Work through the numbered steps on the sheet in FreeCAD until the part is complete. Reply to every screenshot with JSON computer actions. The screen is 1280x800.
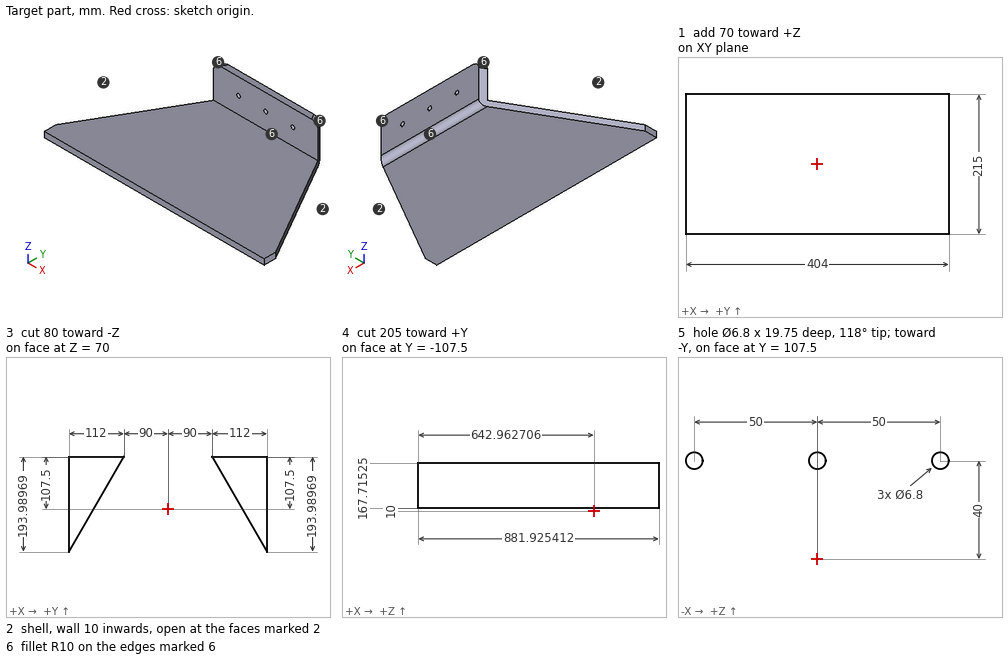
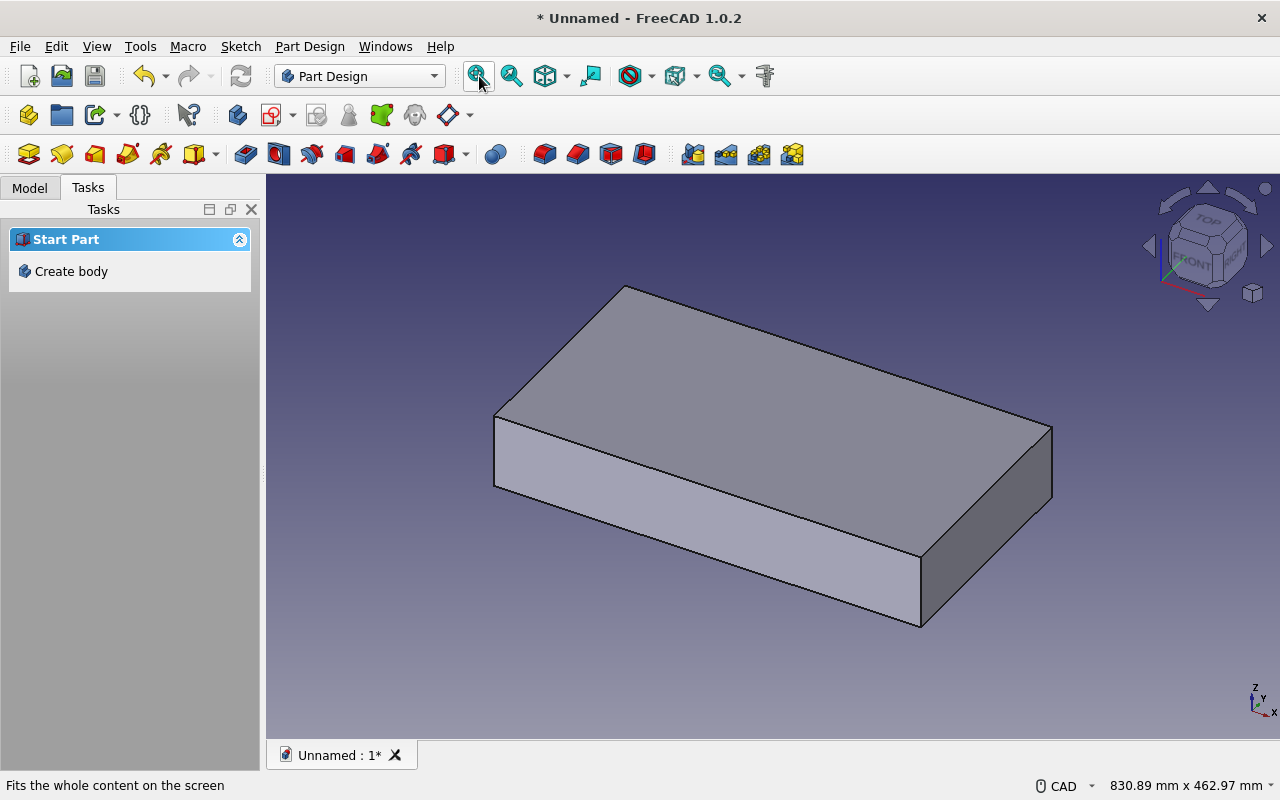
{"action": "left_click", "coordinate": [1024, 489]}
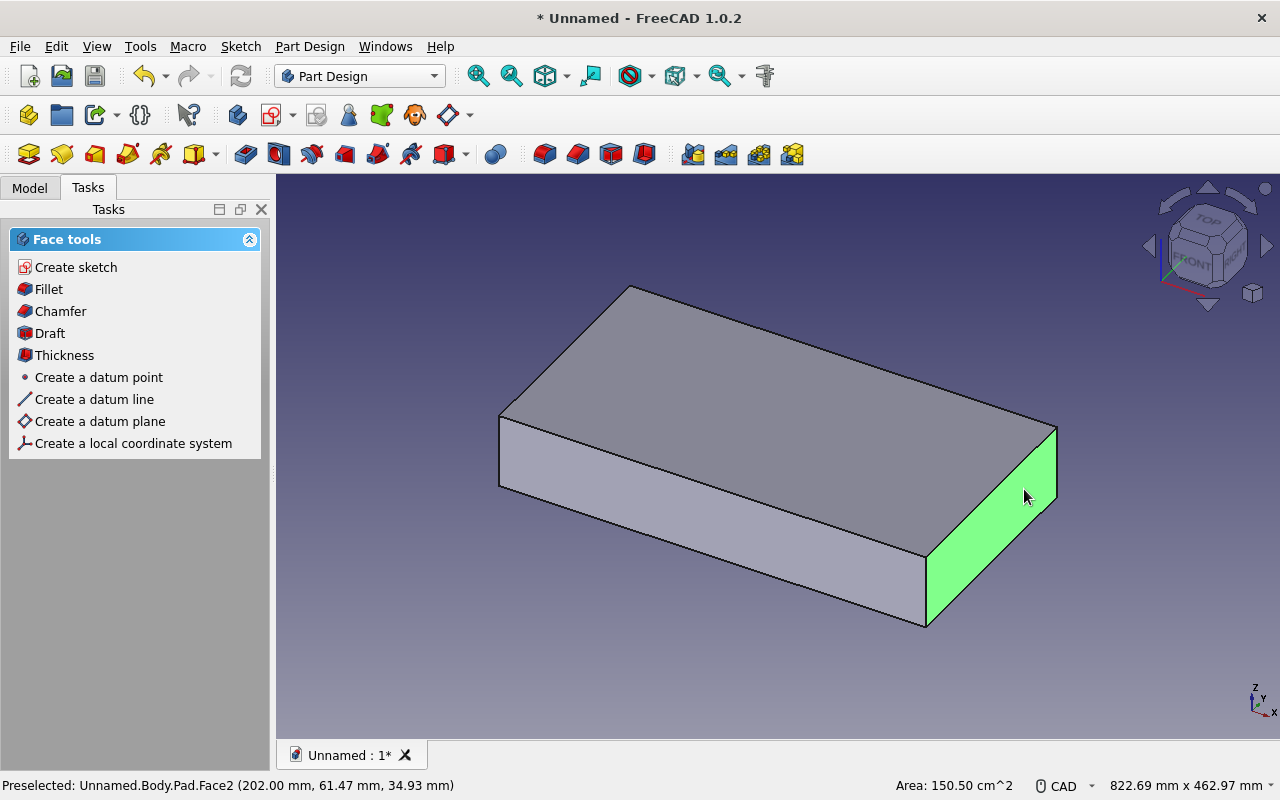
{"action": "key", "text": "0"}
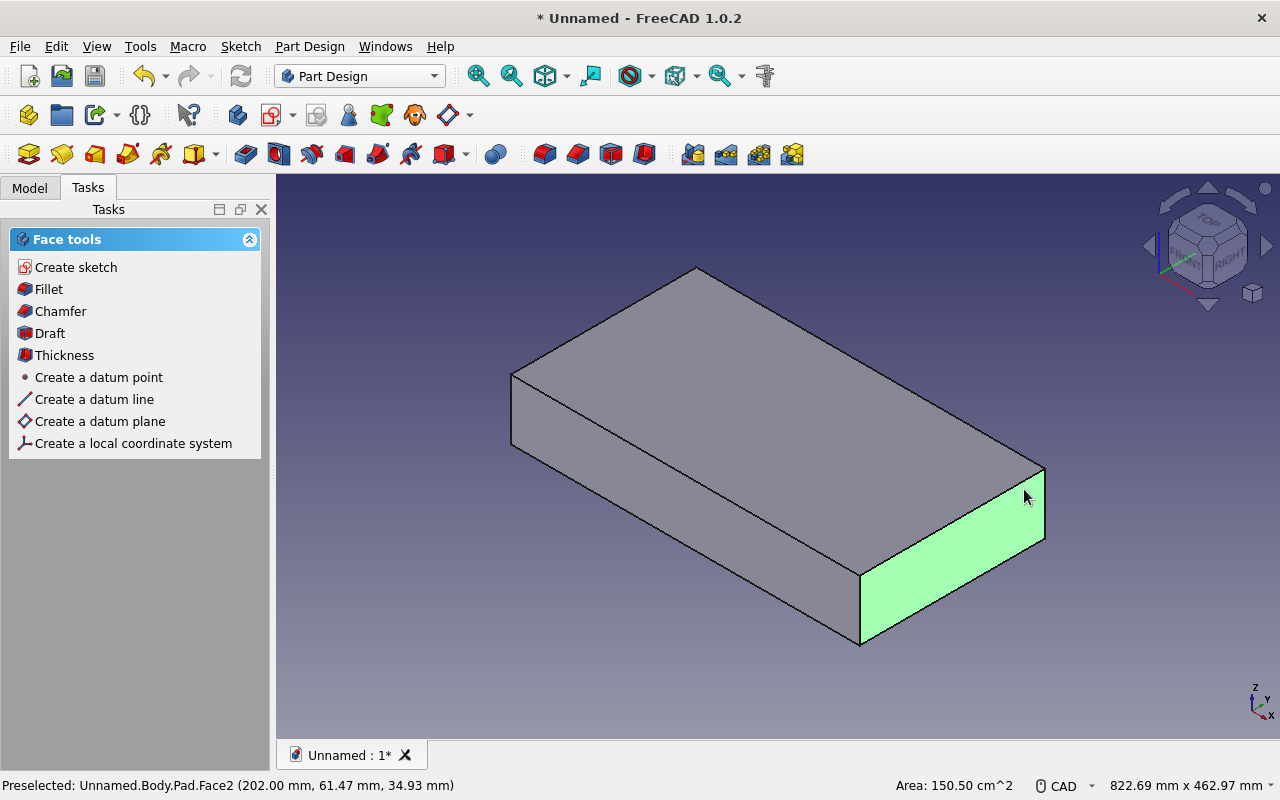
{"action": "key", "text": "2"}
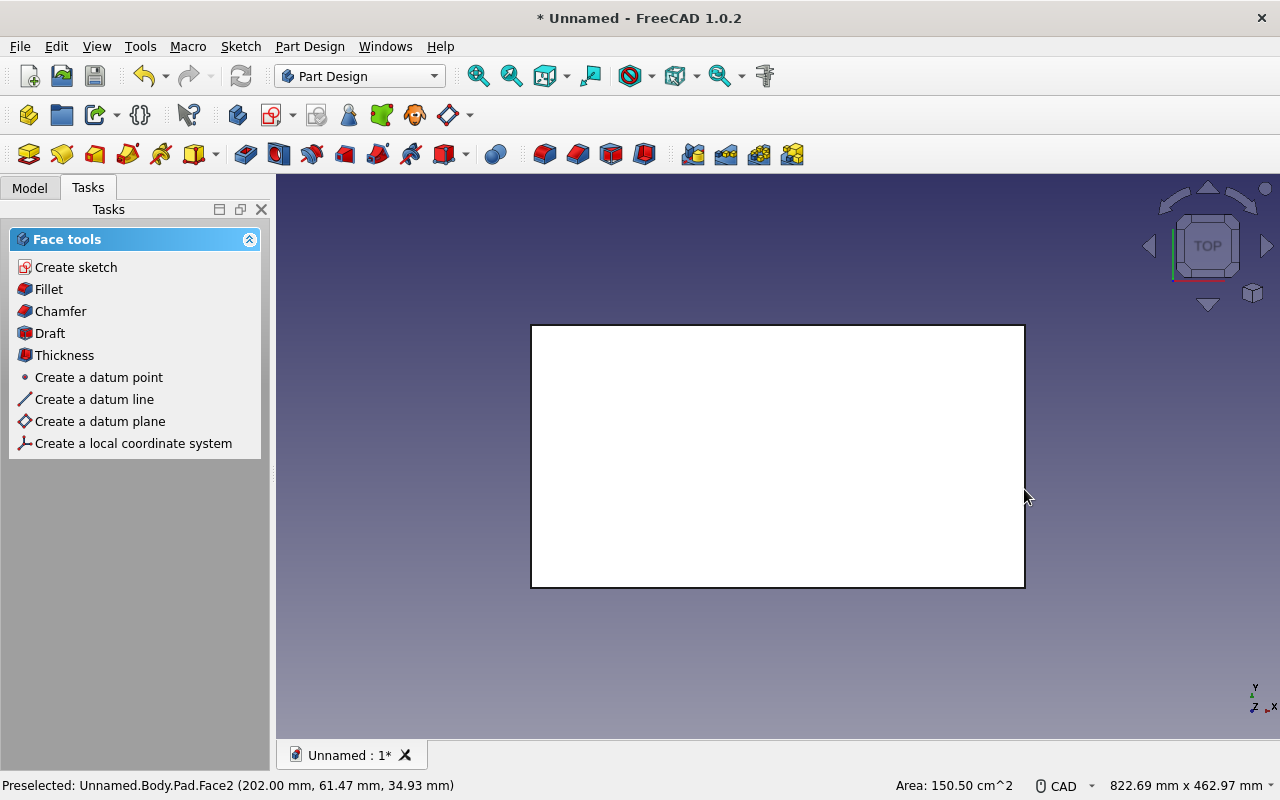
{"action": "key", "text": "1"}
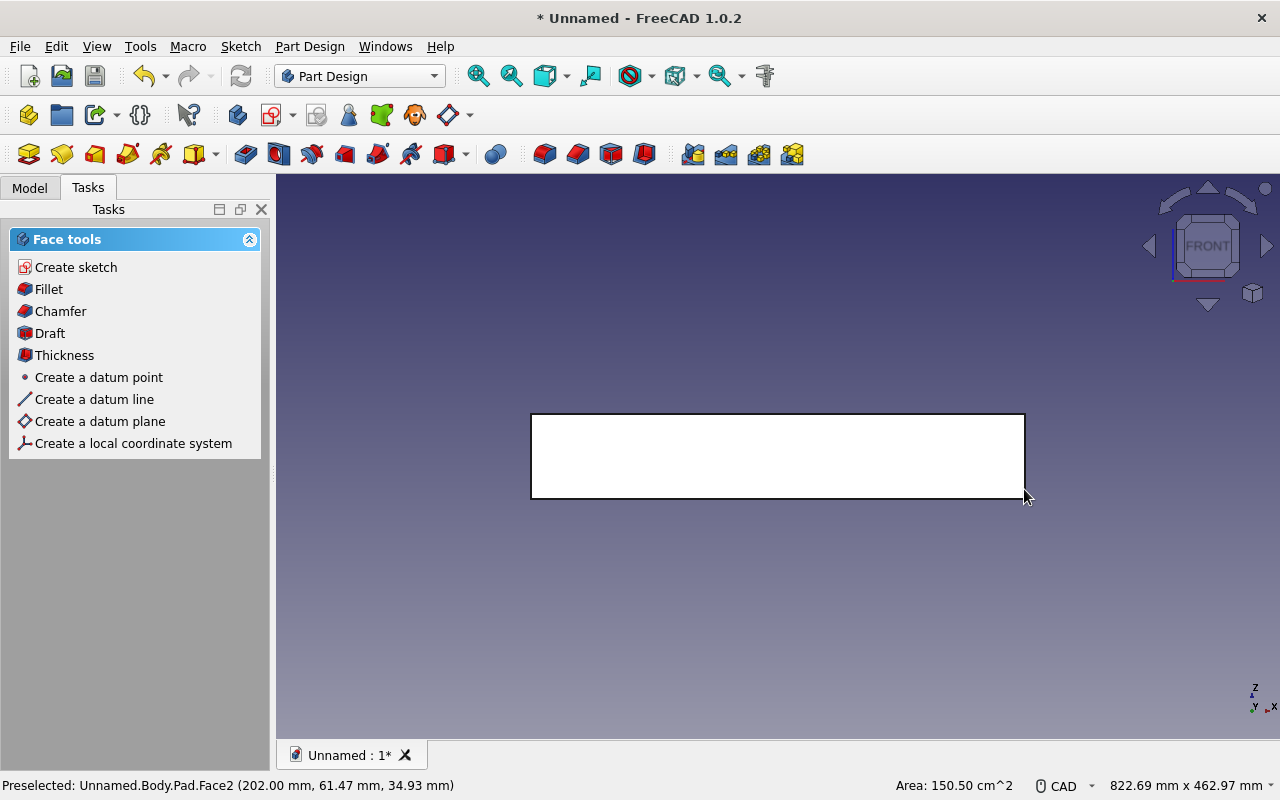
{"action": "key", "text": "3"}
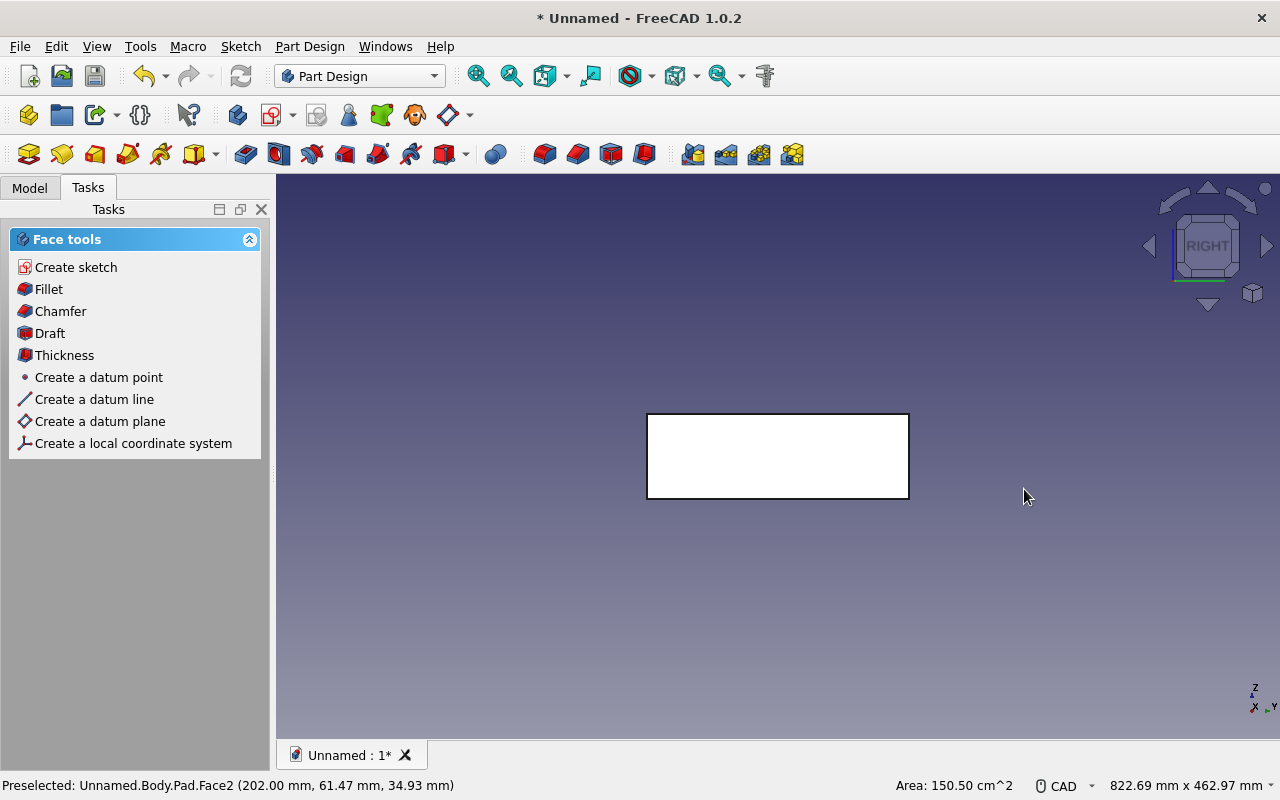
{"action": "left_click", "coordinate": [479, 76]}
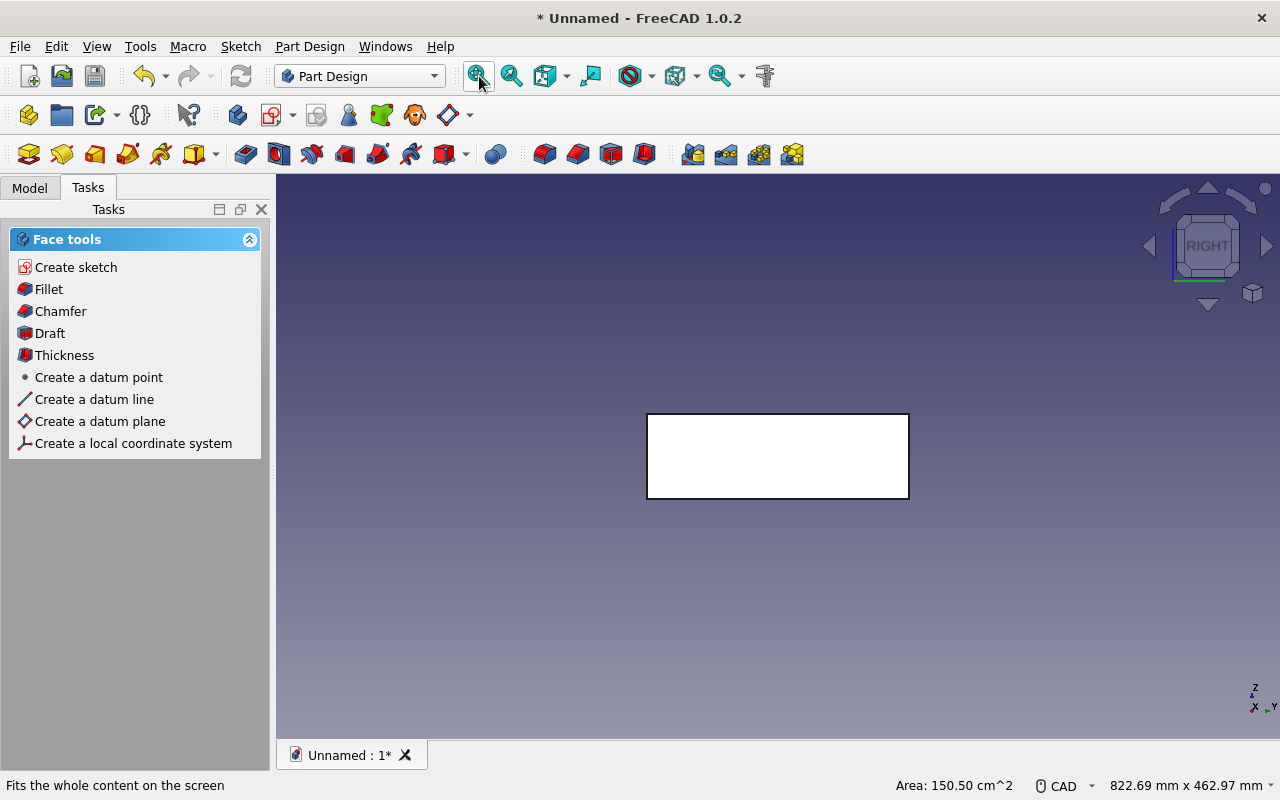
{"action": "key", "text": "5"}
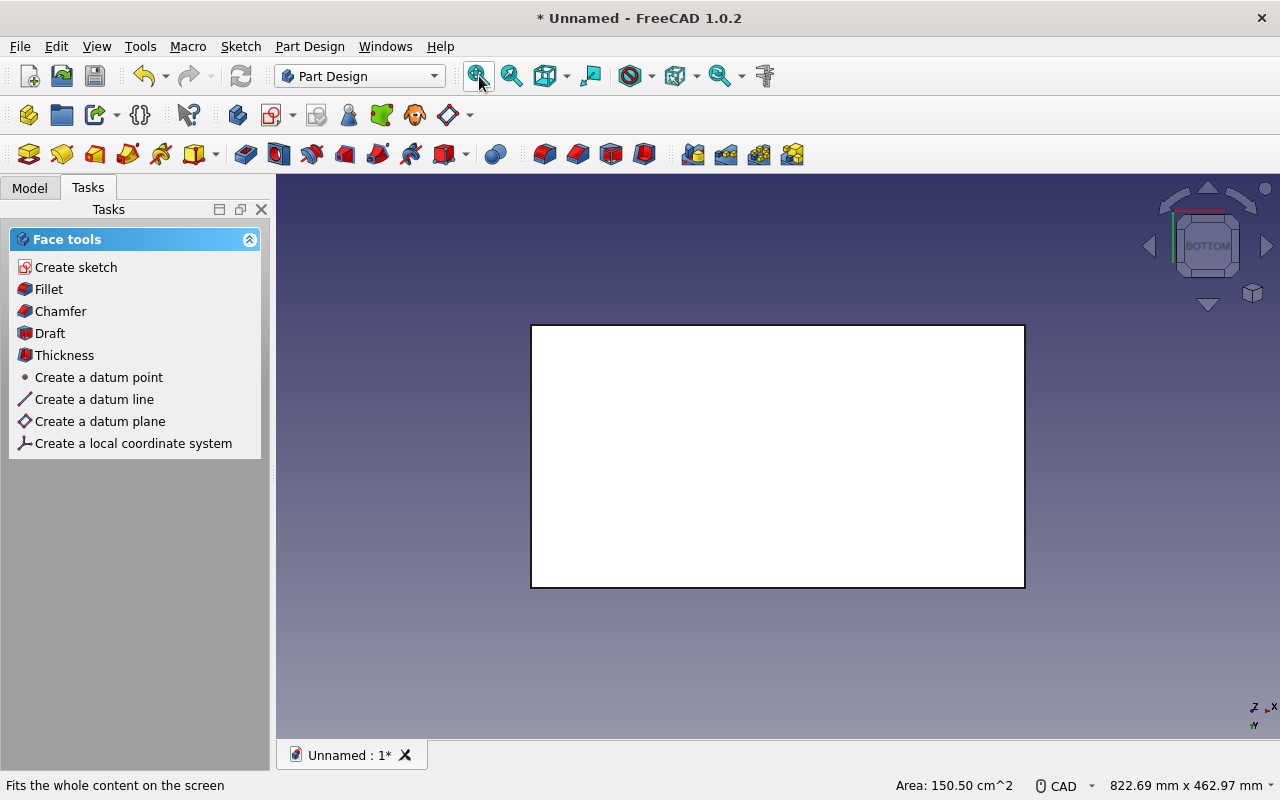
{"action": "key", "text": "4"}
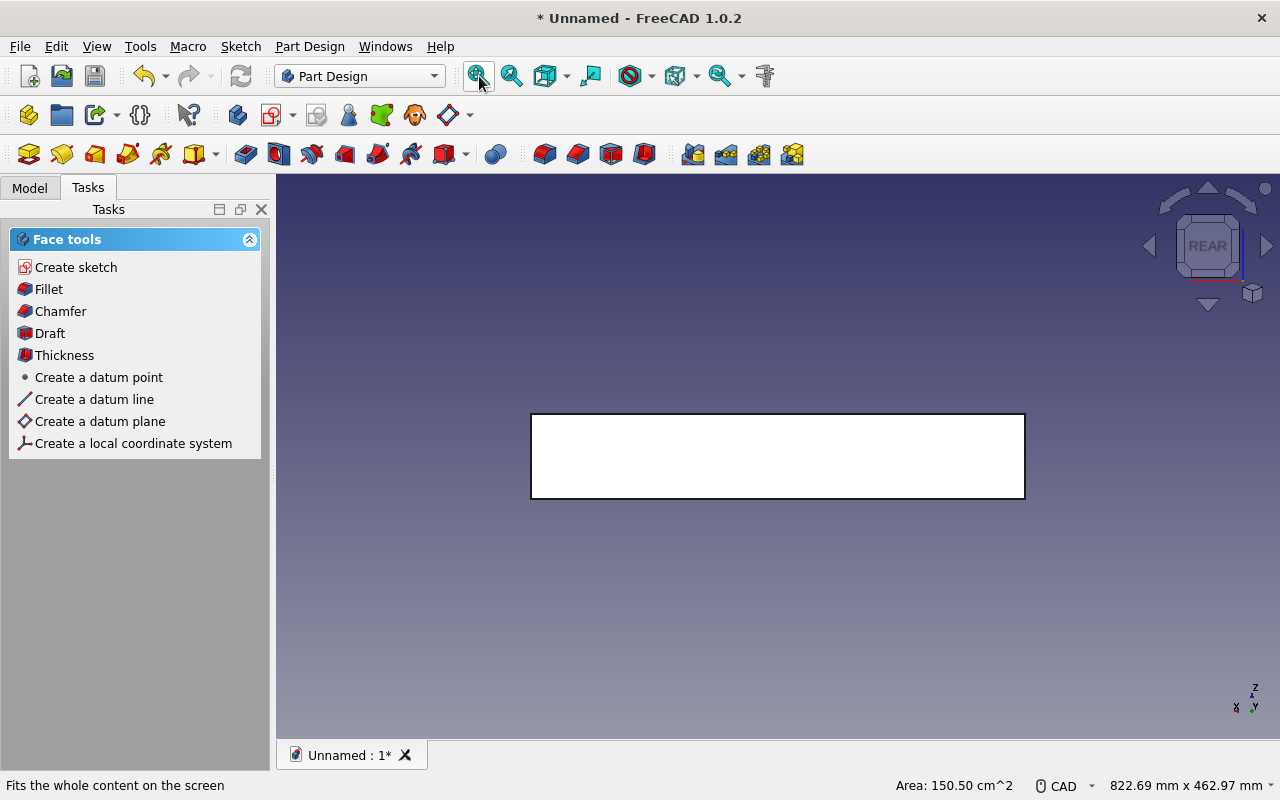
{"action": "key", "text": "6"}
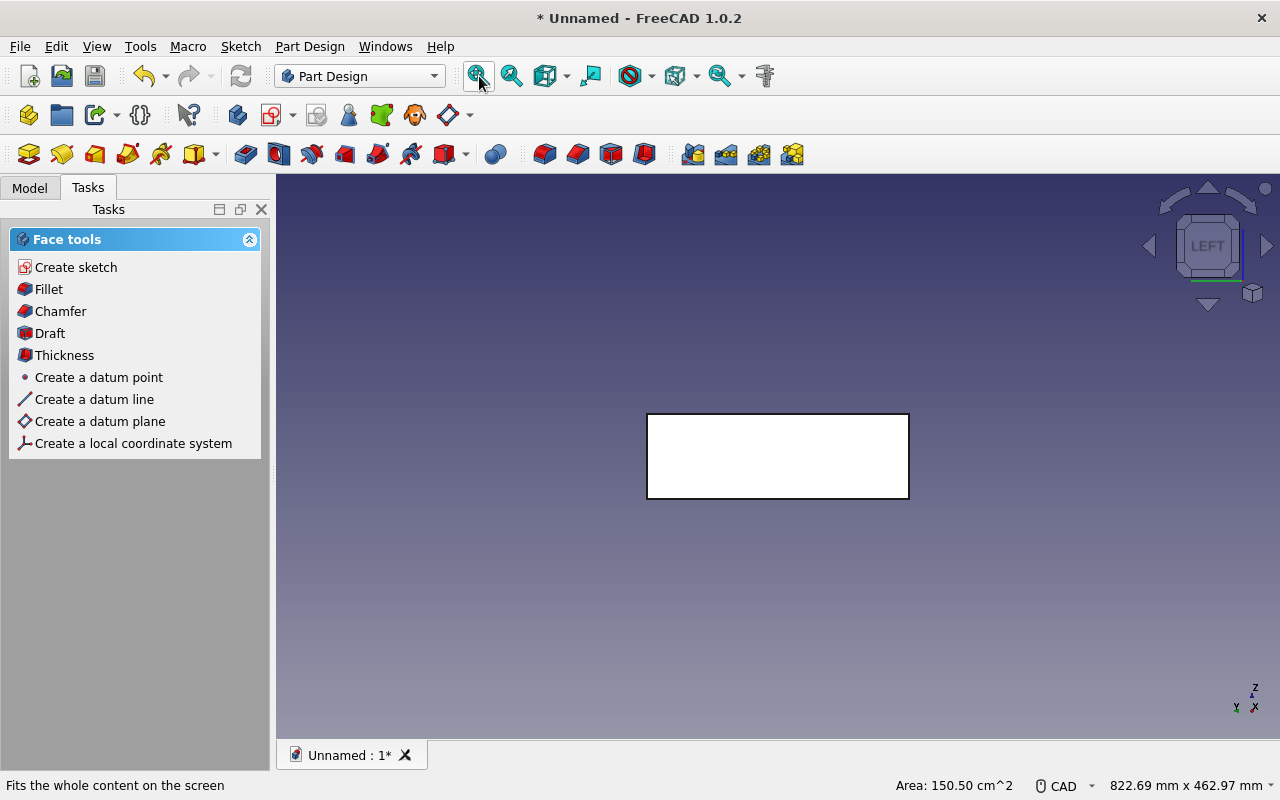
{"action": "left_click", "coordinate": [479, 76]}